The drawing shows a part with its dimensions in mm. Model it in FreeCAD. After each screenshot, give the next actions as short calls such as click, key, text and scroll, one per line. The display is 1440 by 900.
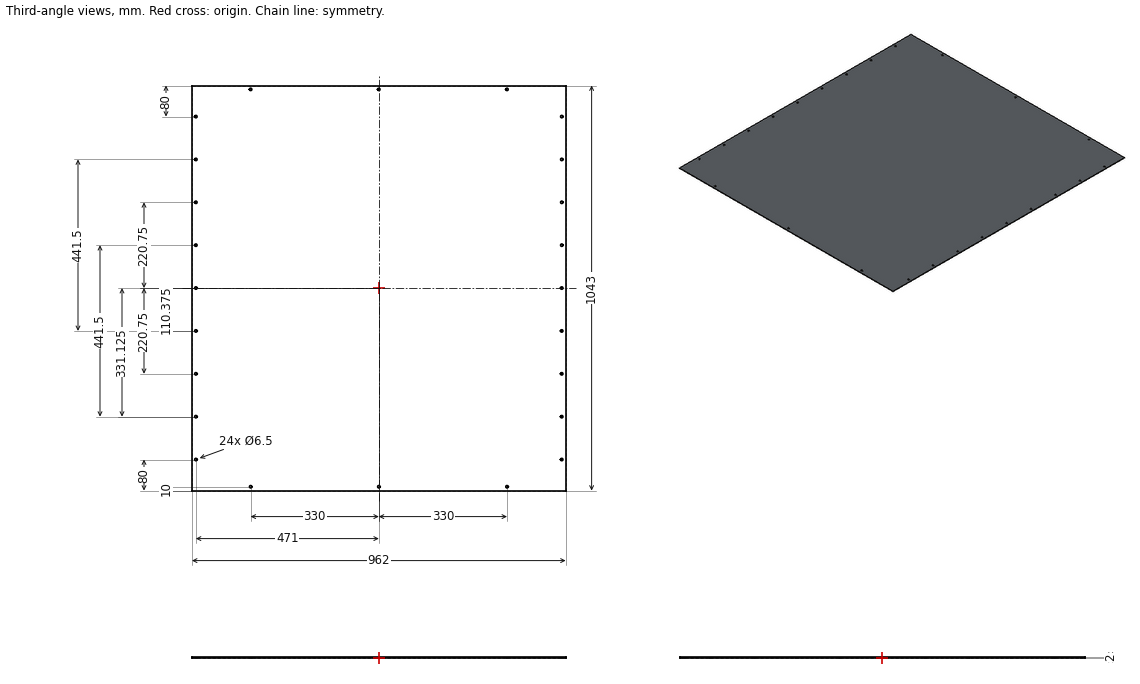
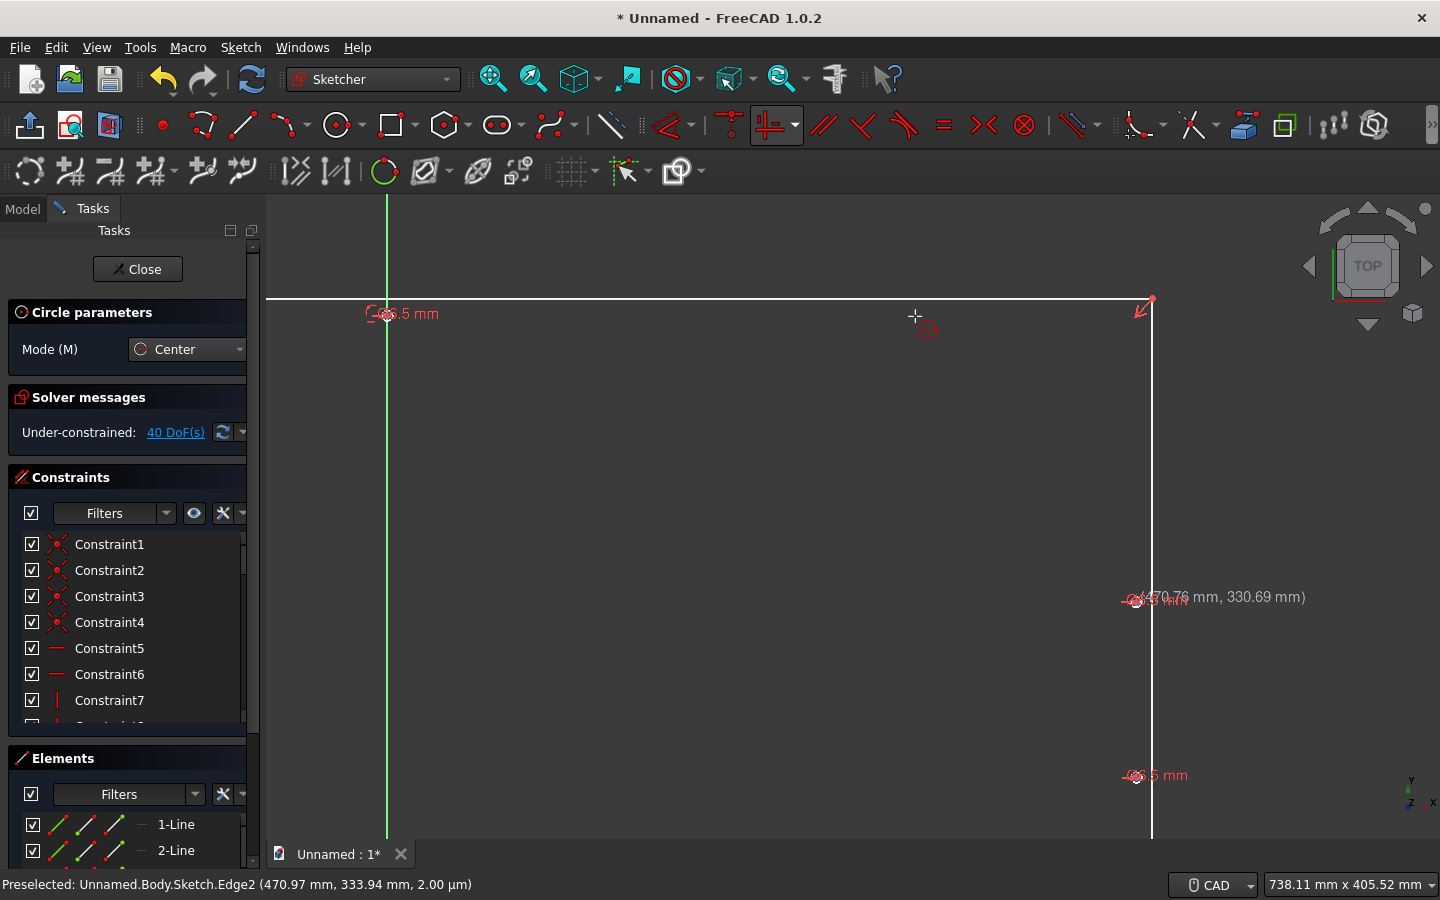
click(912, 315)
move(916, 318)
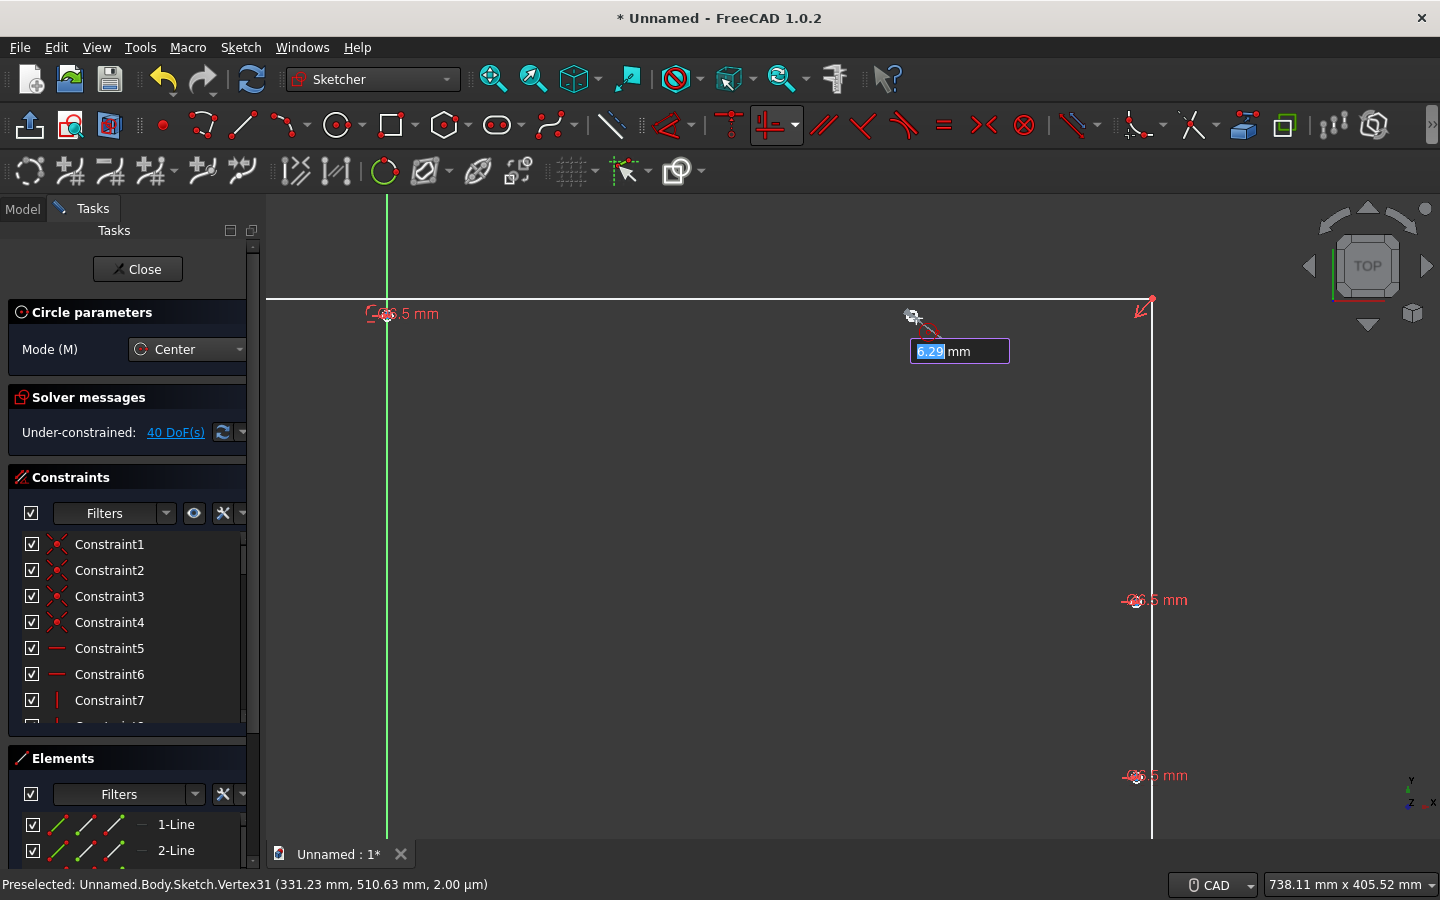
text(6.5)
key(Return)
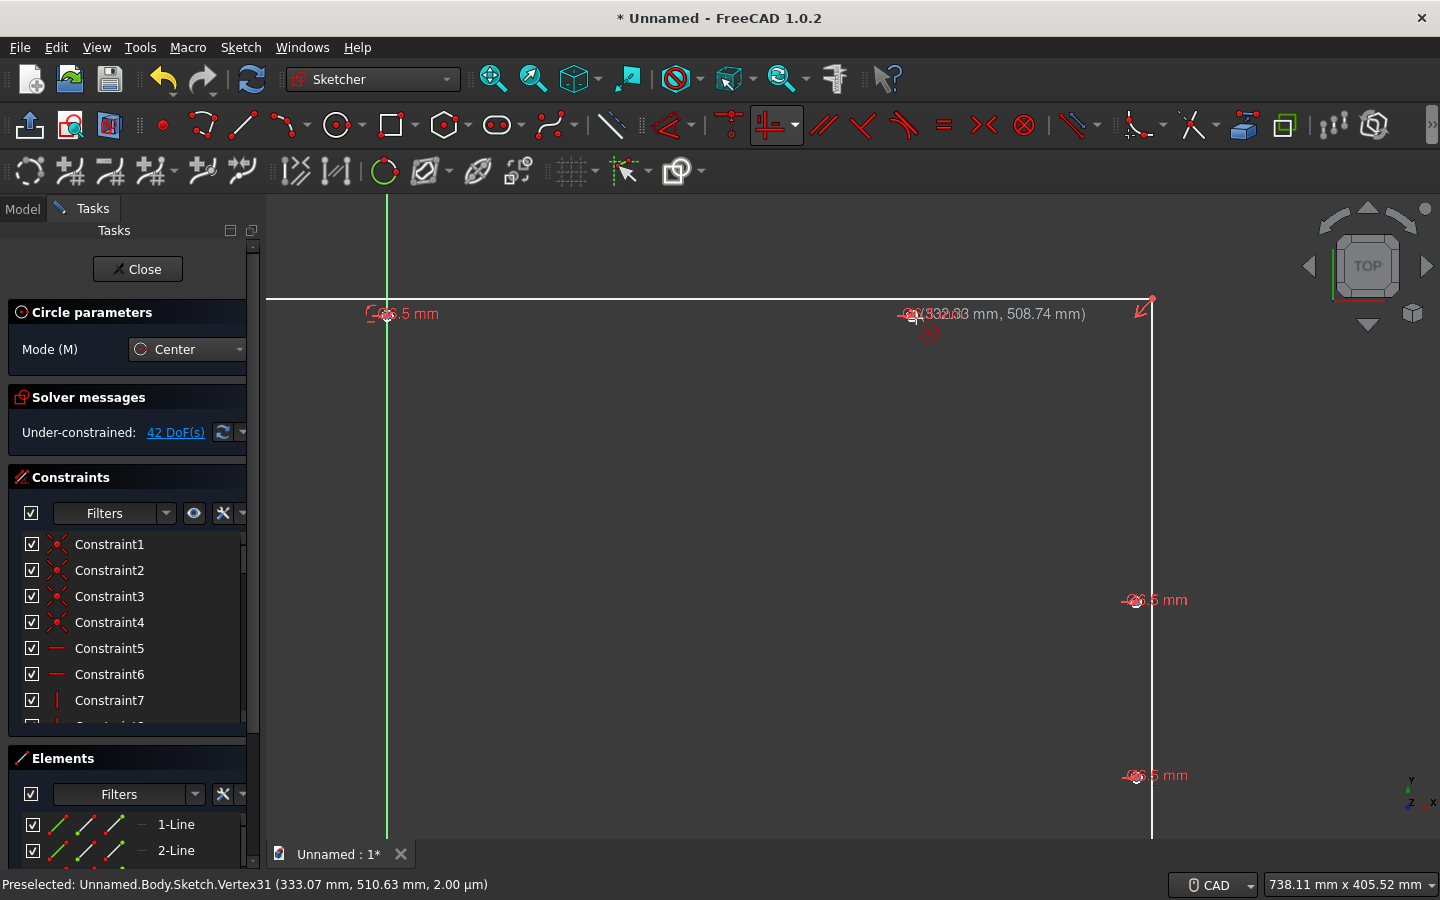
scroll(1137, 426, up, 8)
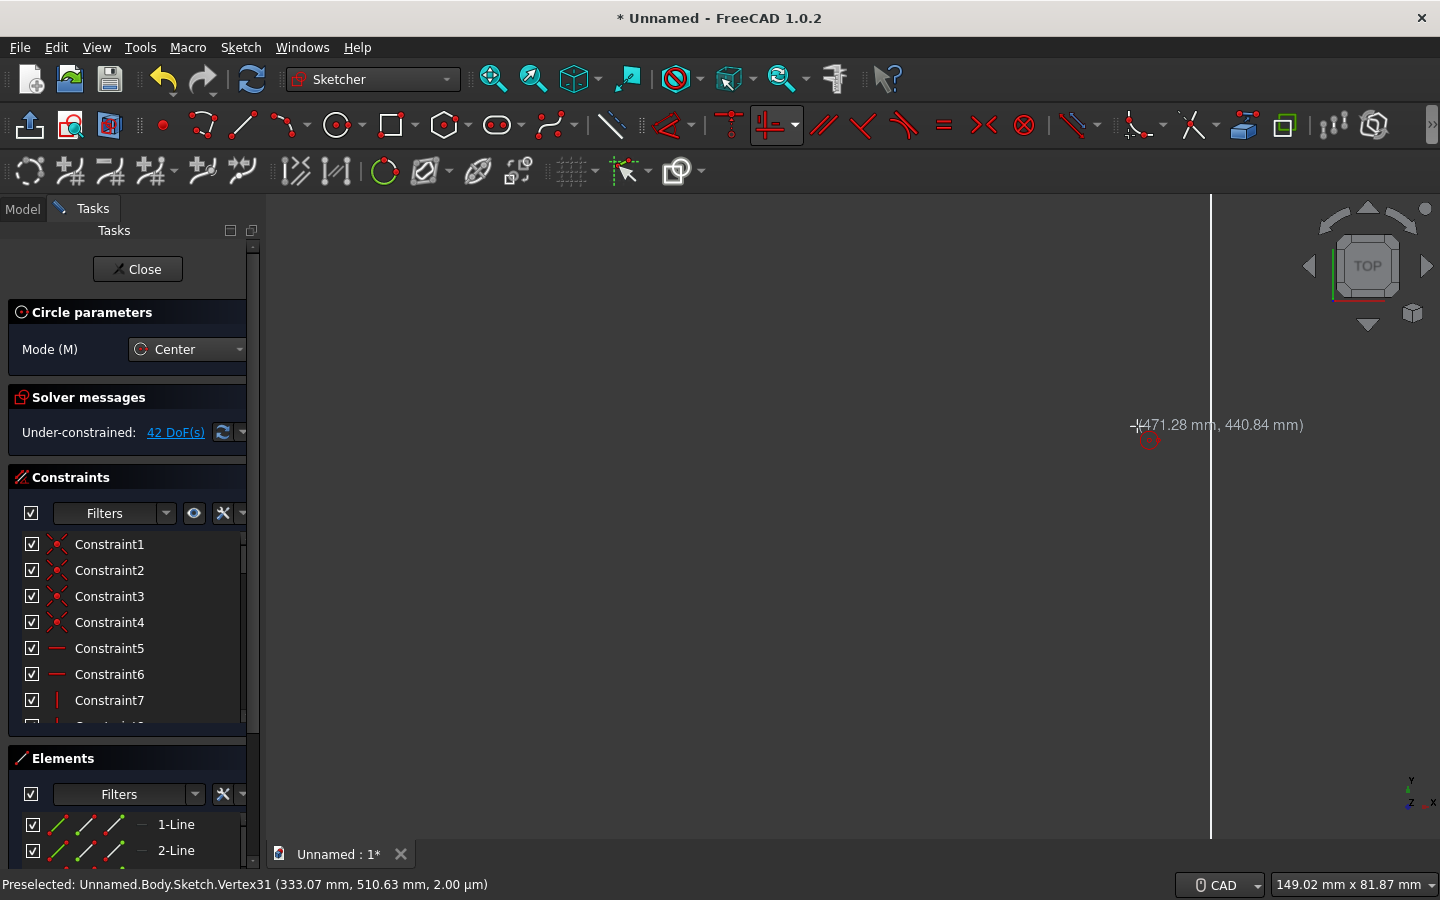
scroll(961, 339, down, 15)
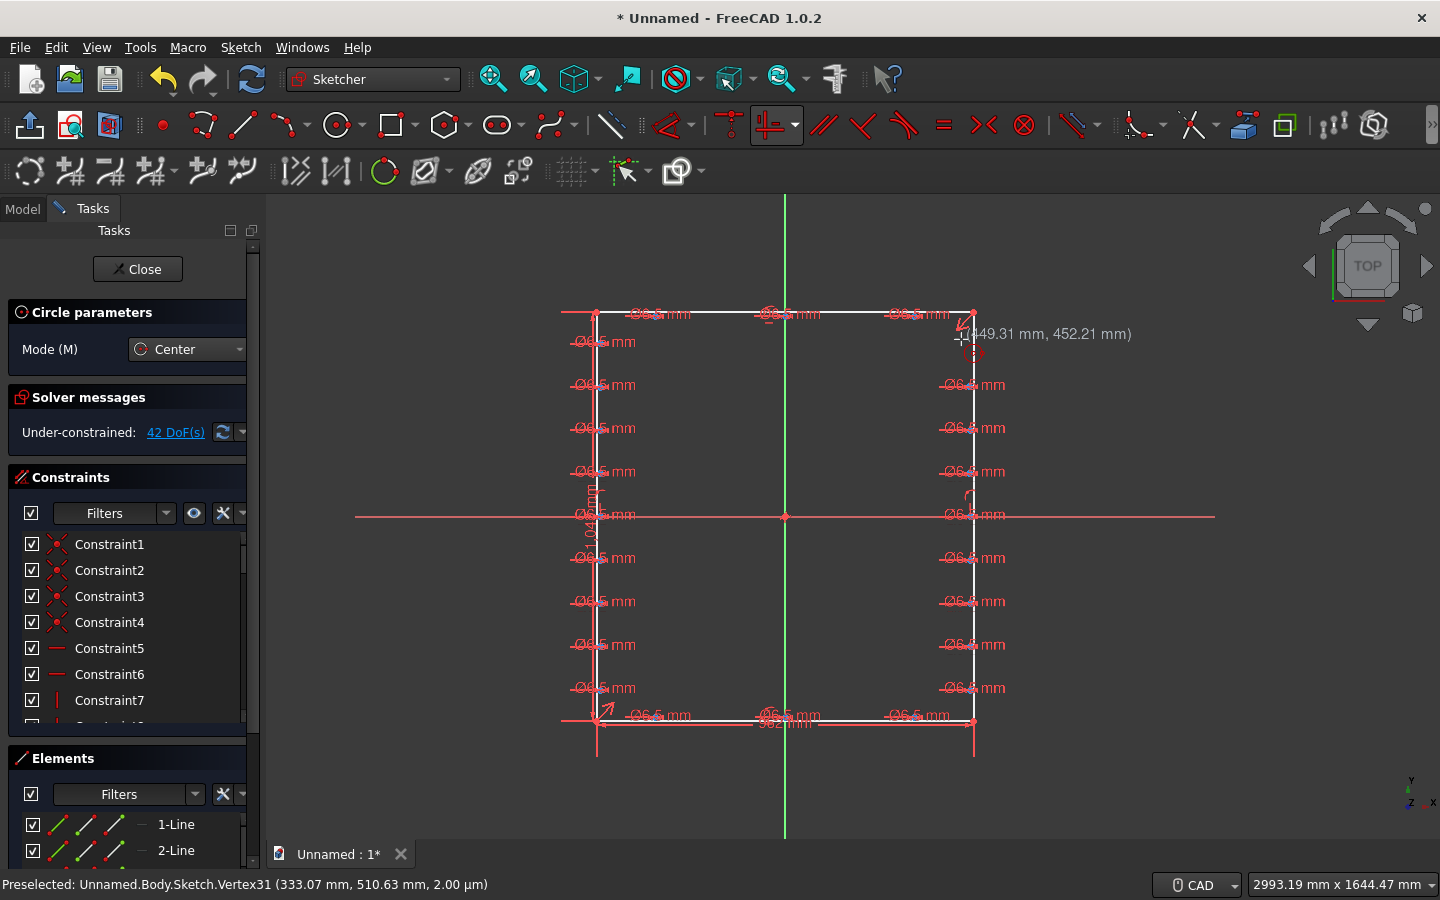
scroll(970, 343, up, 7)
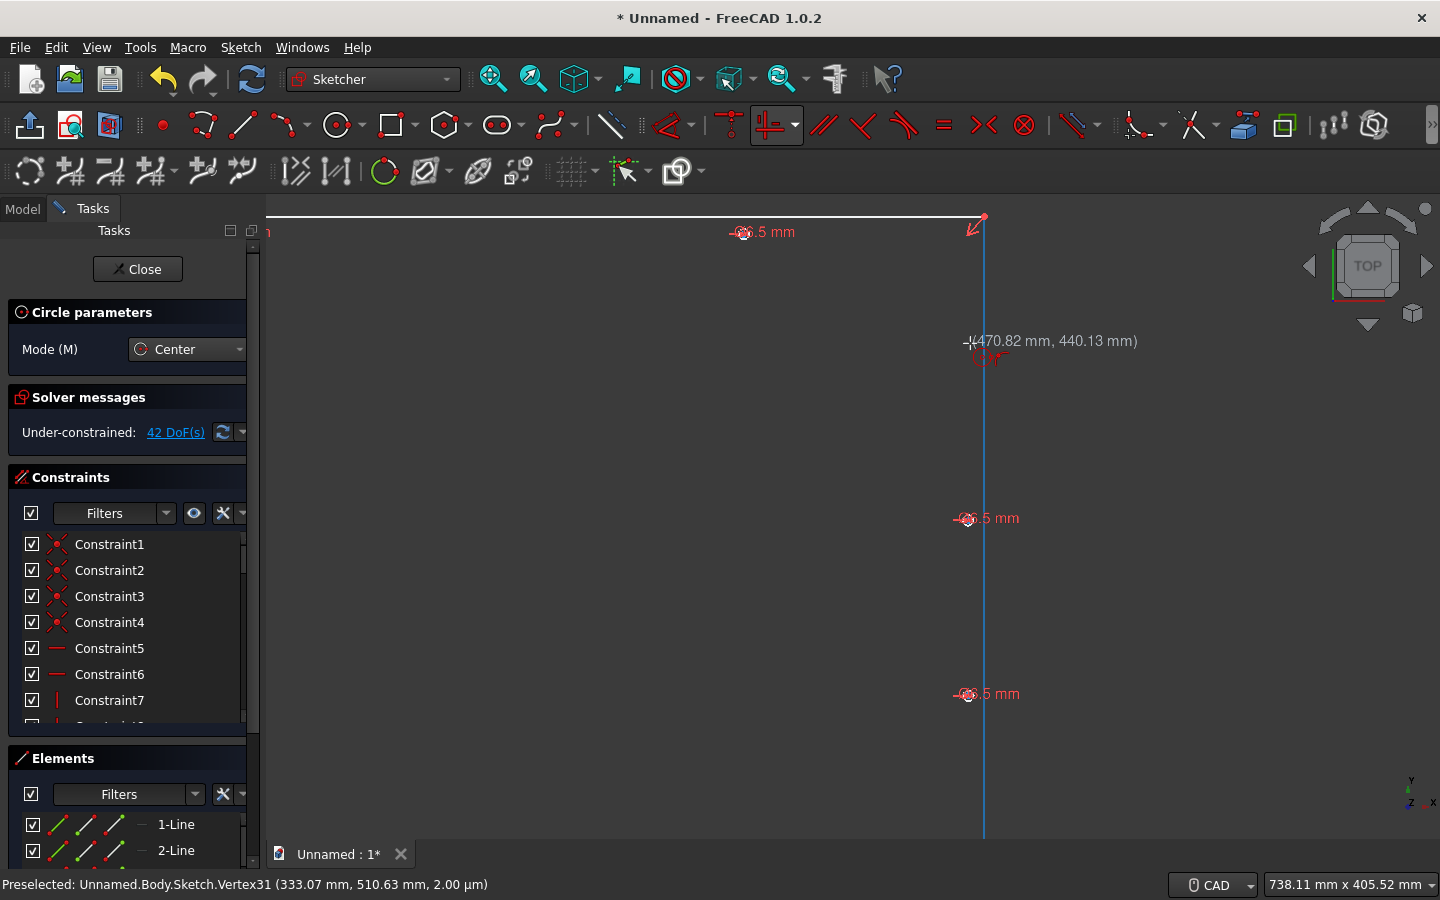
click(968, 344)
move(965, 341)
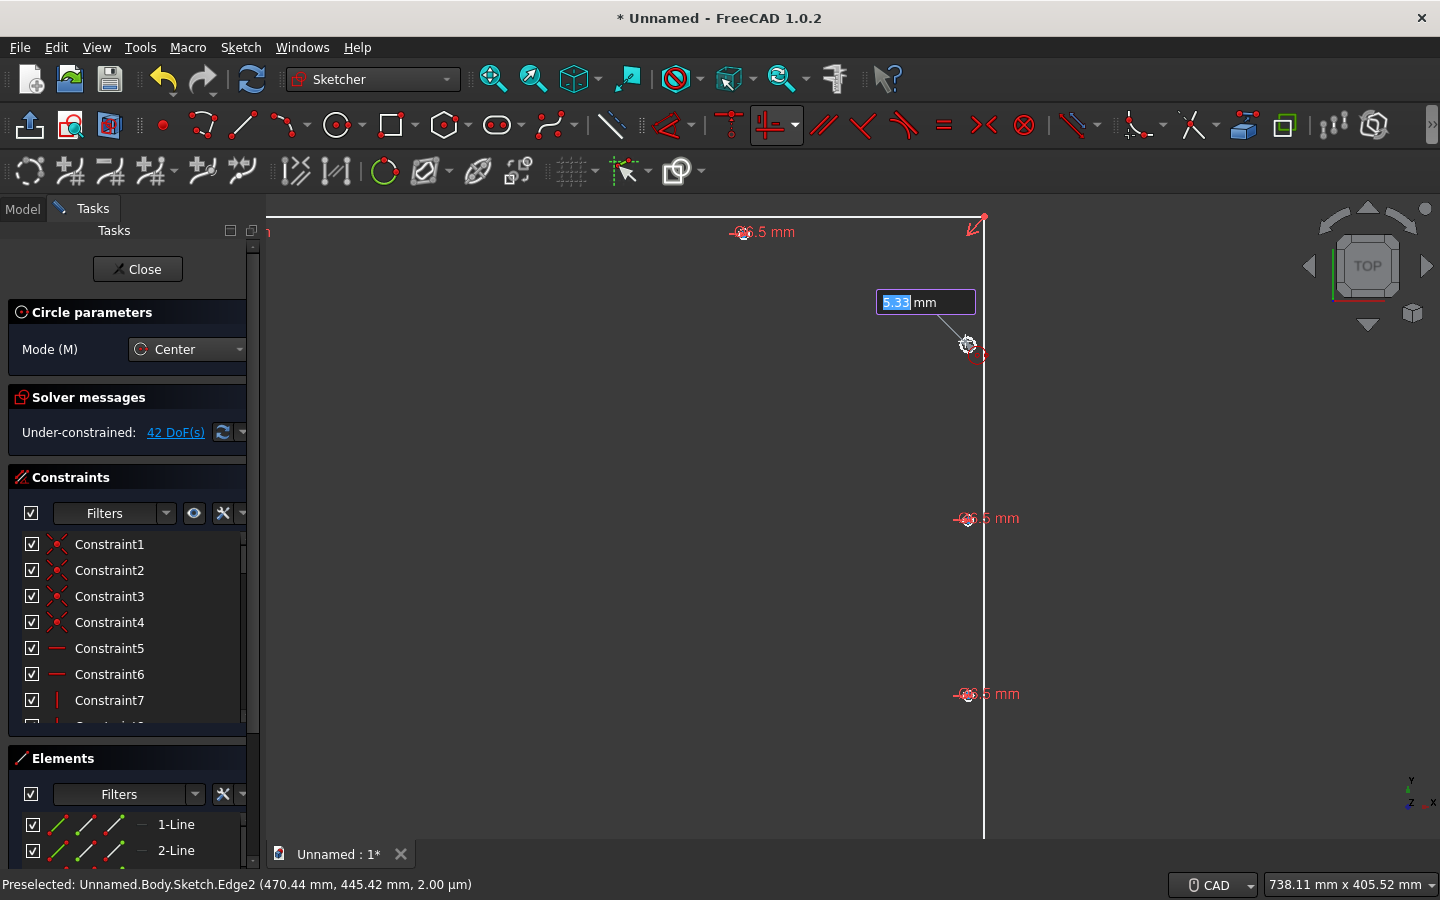
text(6.5)
key(Return)
key(Escape)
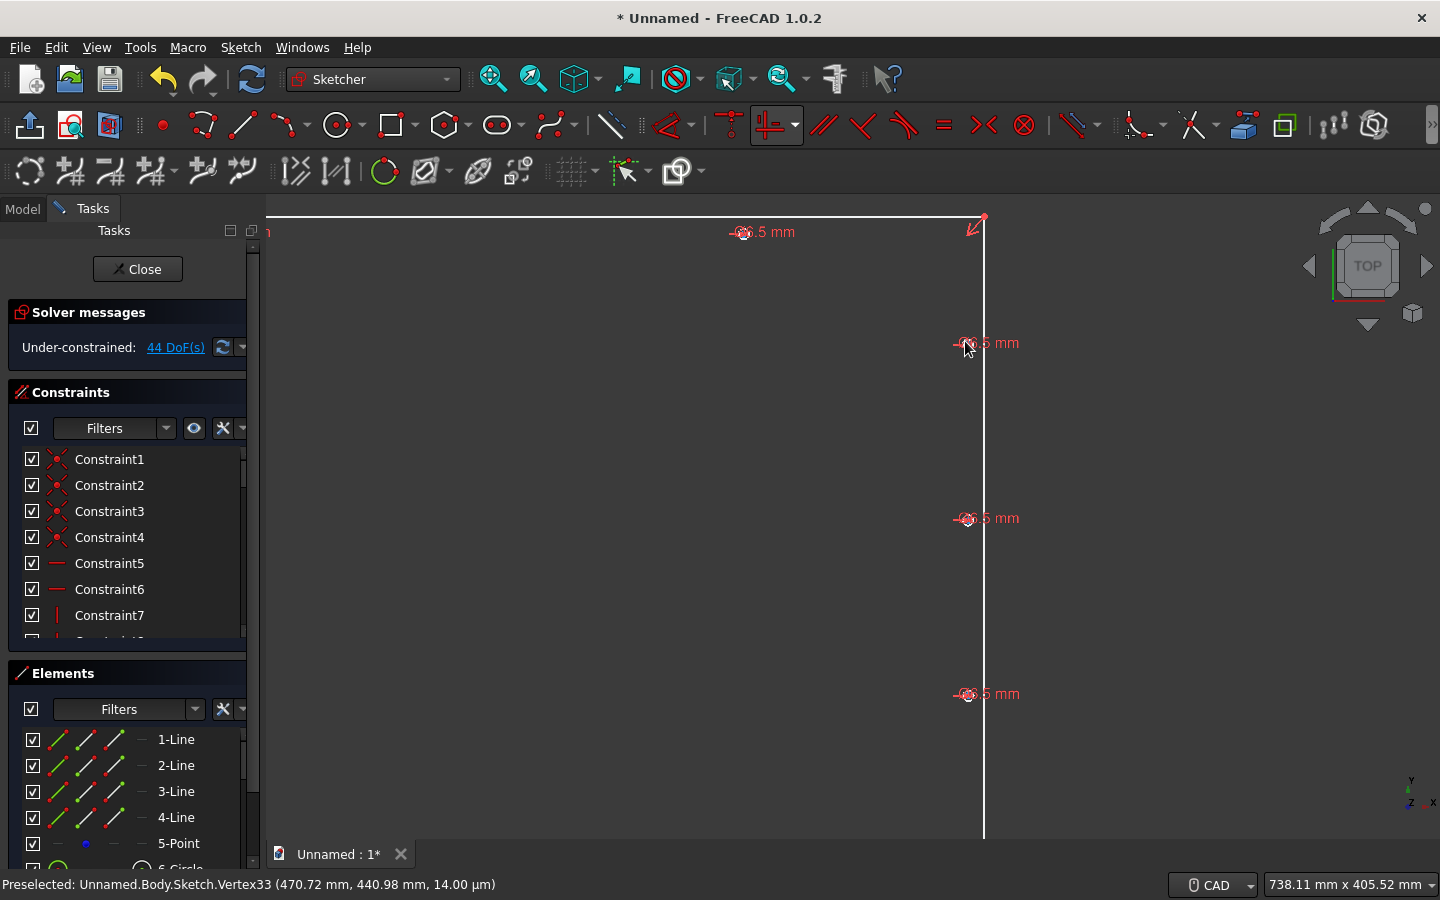
scroll(969, 343, down, 7)